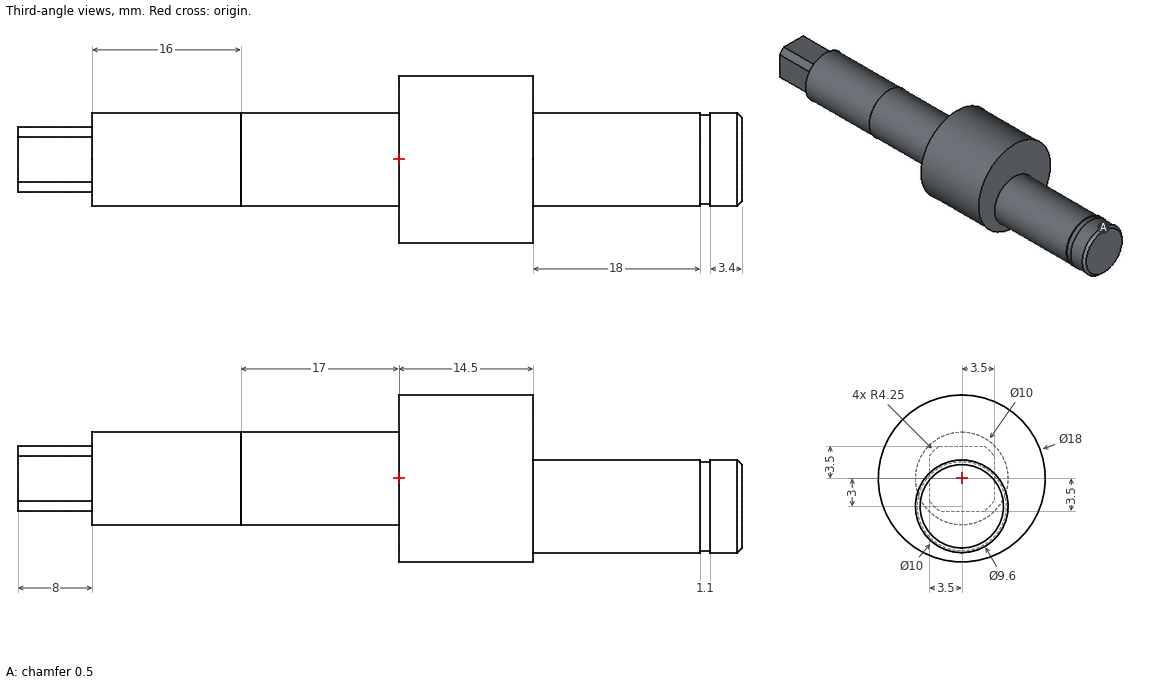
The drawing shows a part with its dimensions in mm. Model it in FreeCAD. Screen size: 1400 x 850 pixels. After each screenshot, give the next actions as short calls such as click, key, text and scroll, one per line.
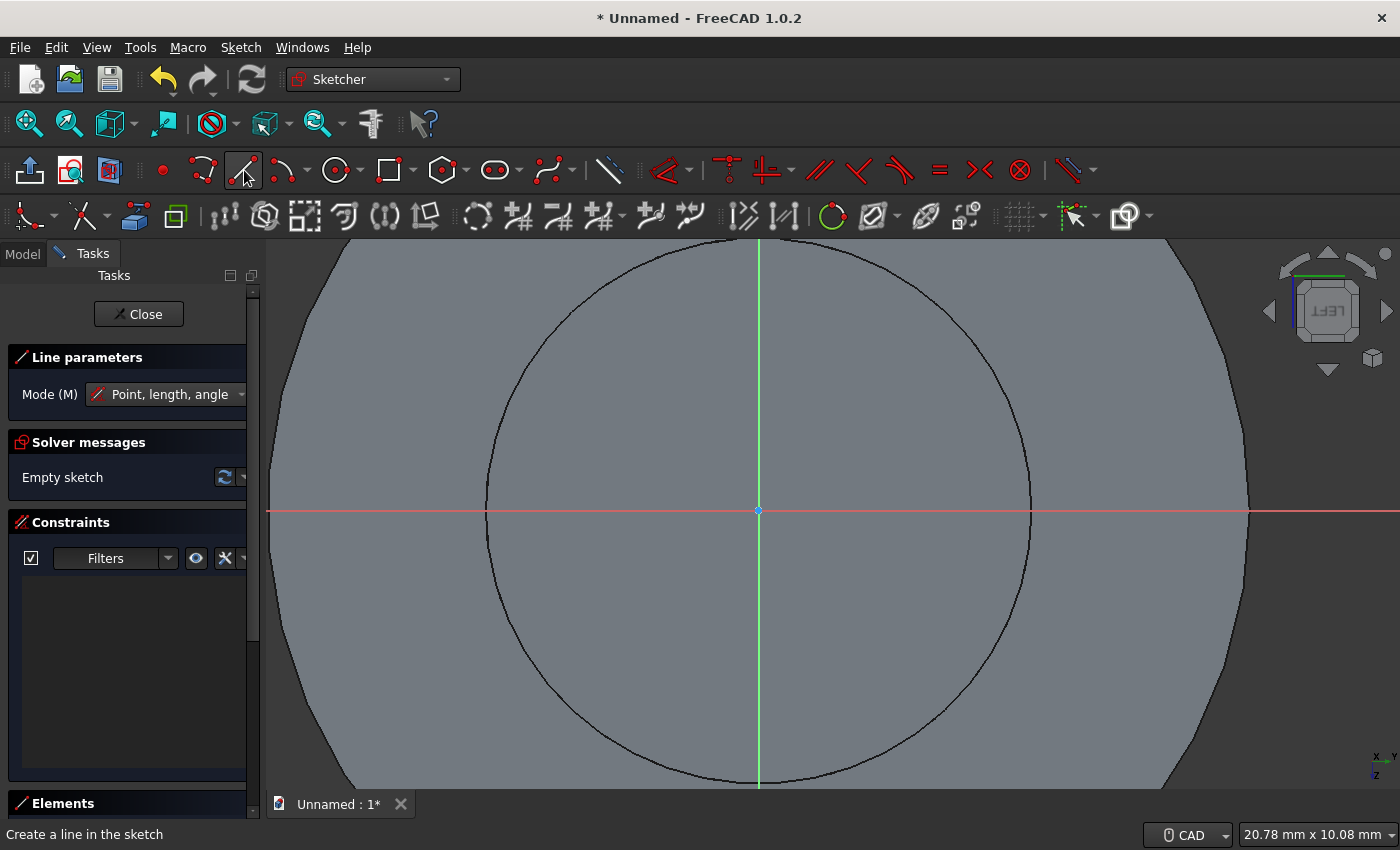
click(568, 379)
click(568, 642)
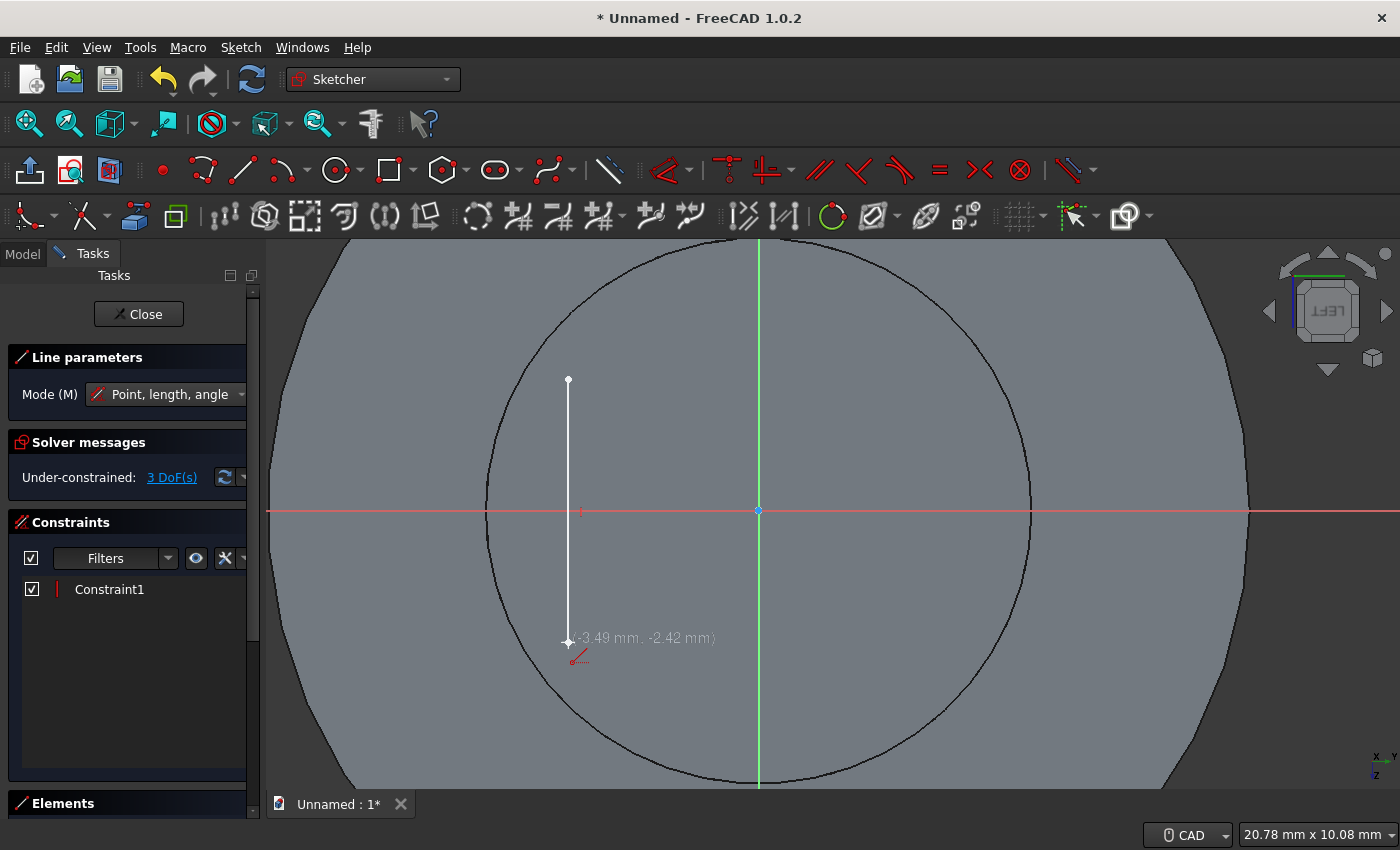
click(627, 702)
click(890, 702)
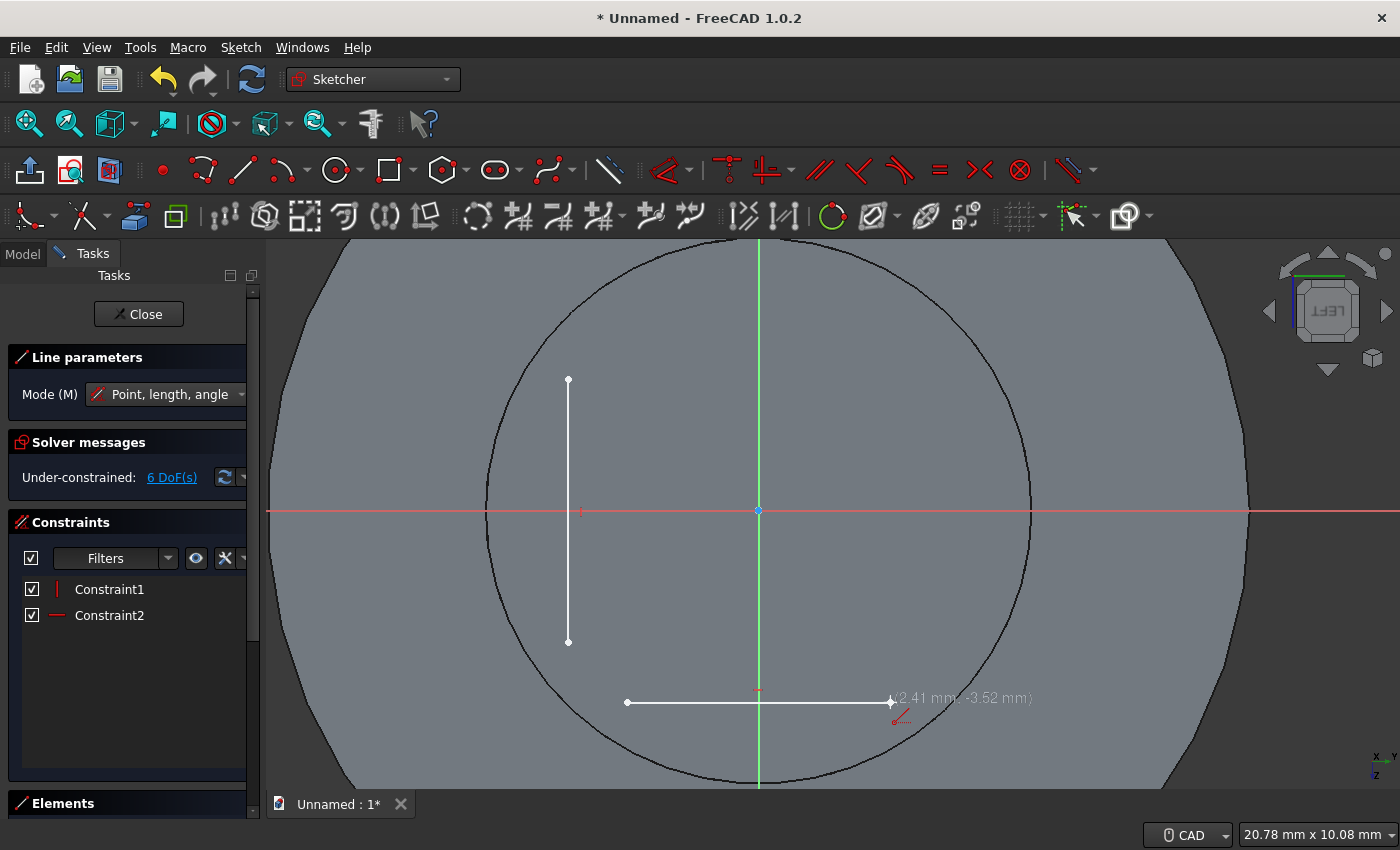
click(950, 642)
click(950, 379)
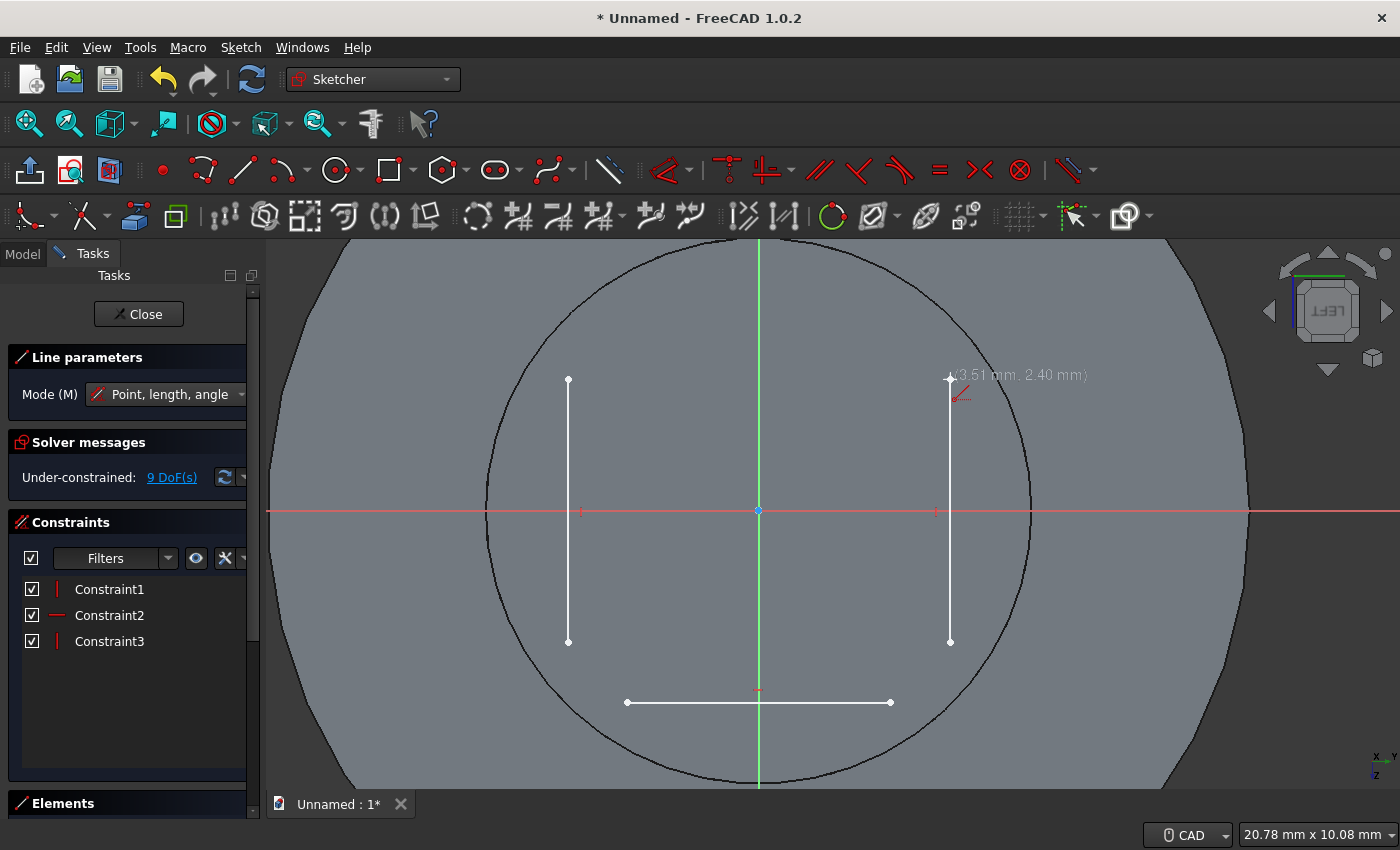
click(890, 320)
click(627, 320)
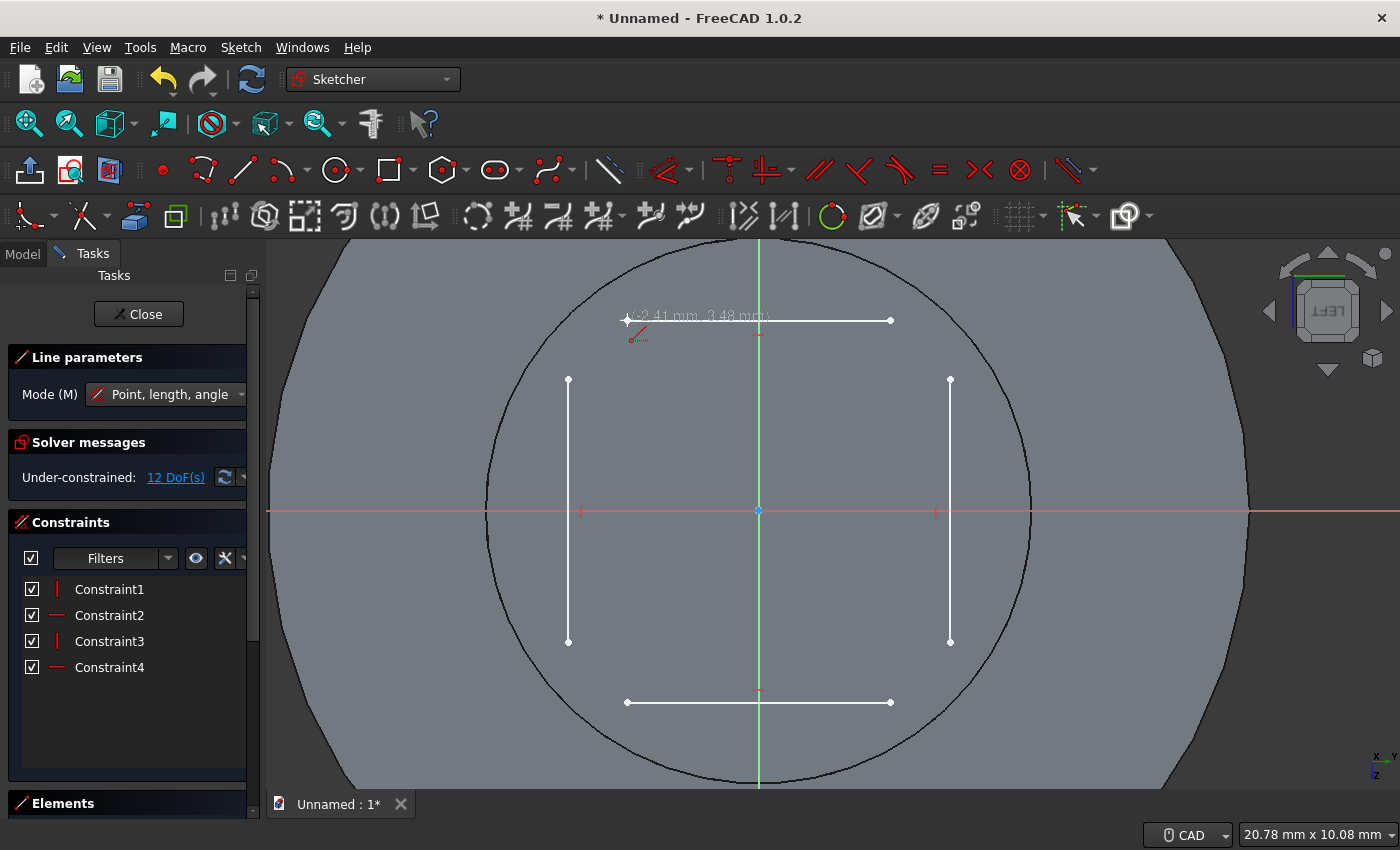
click(310, 170)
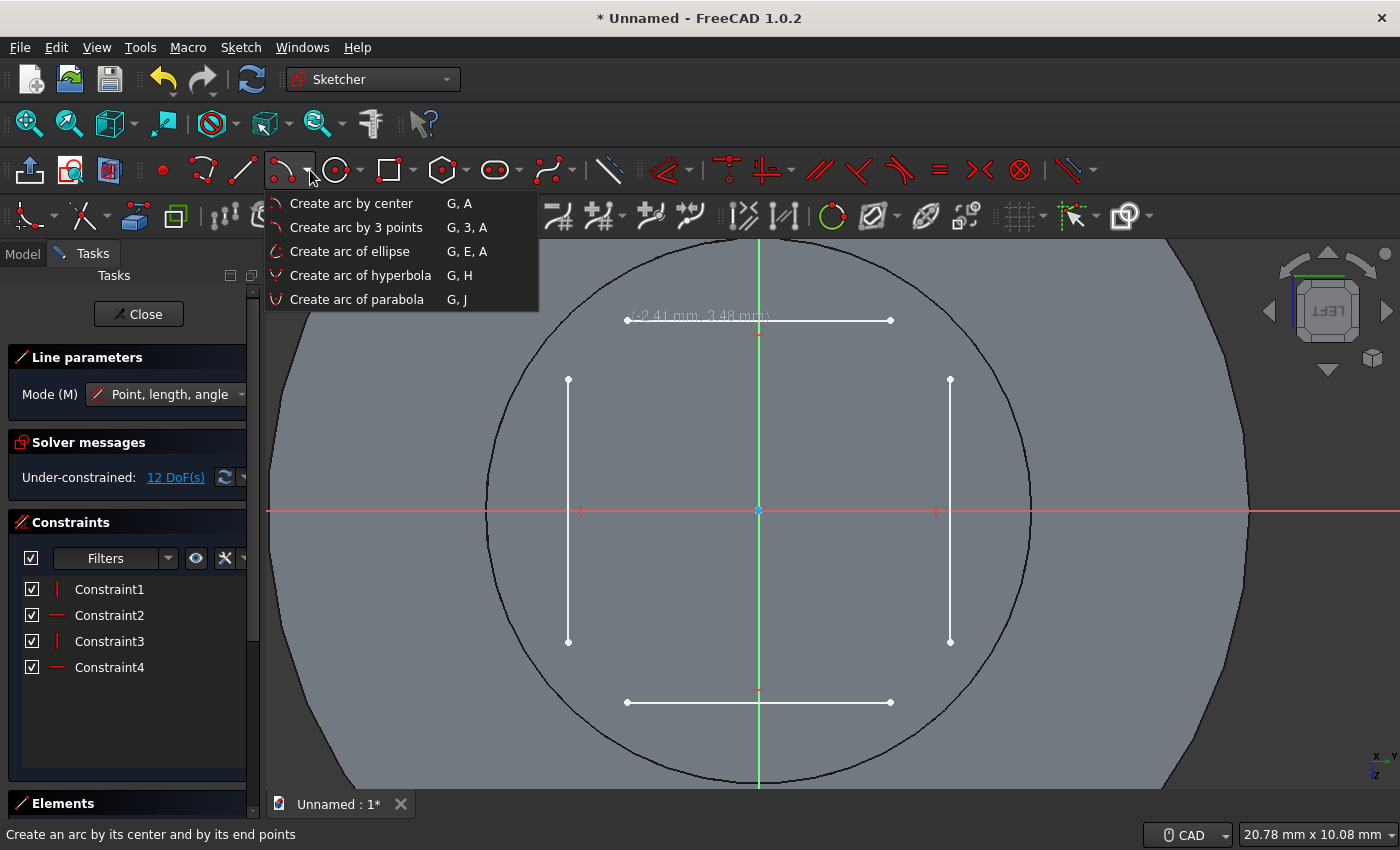
click(402, 227)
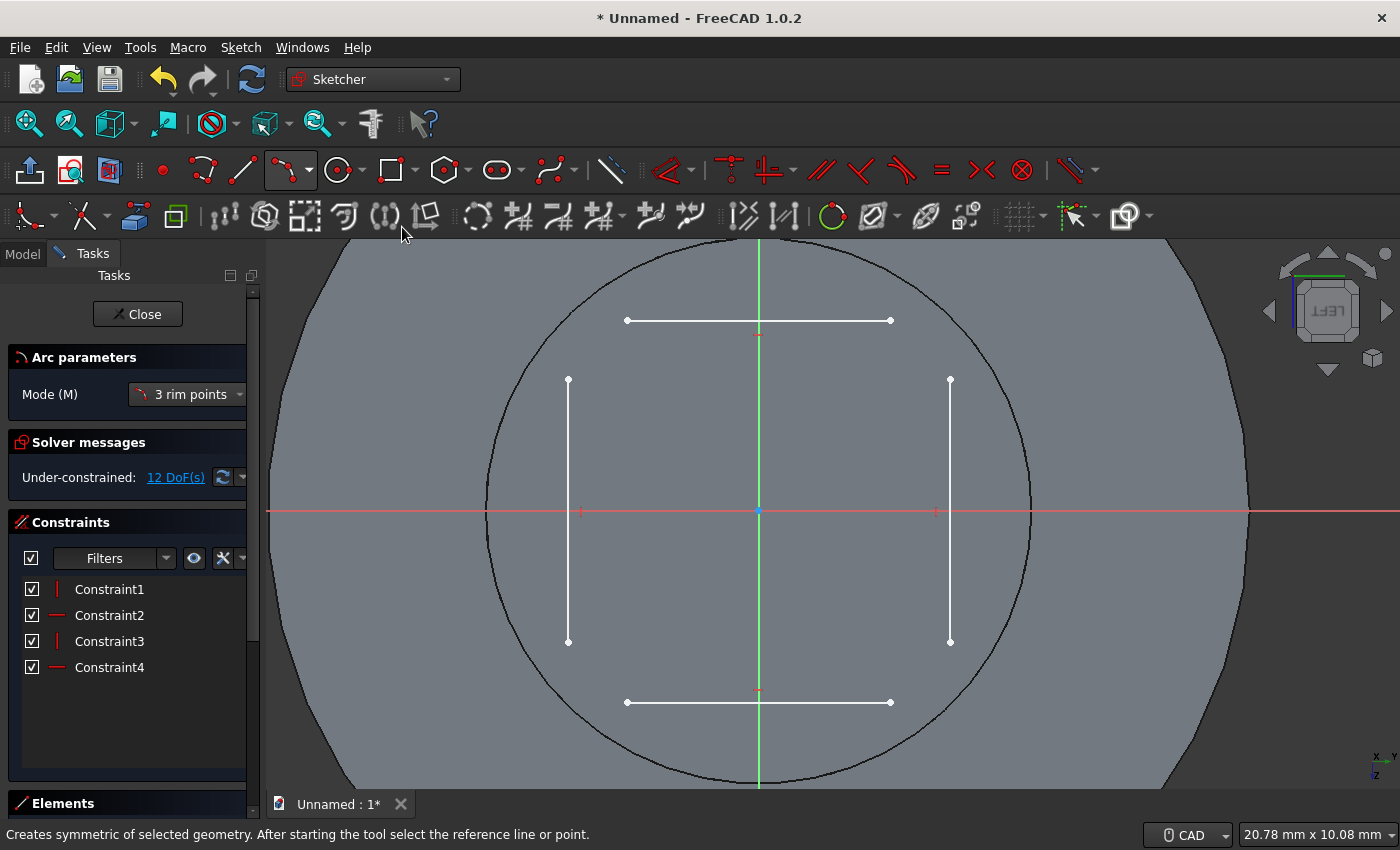
click(568, 643)
click(627, 703)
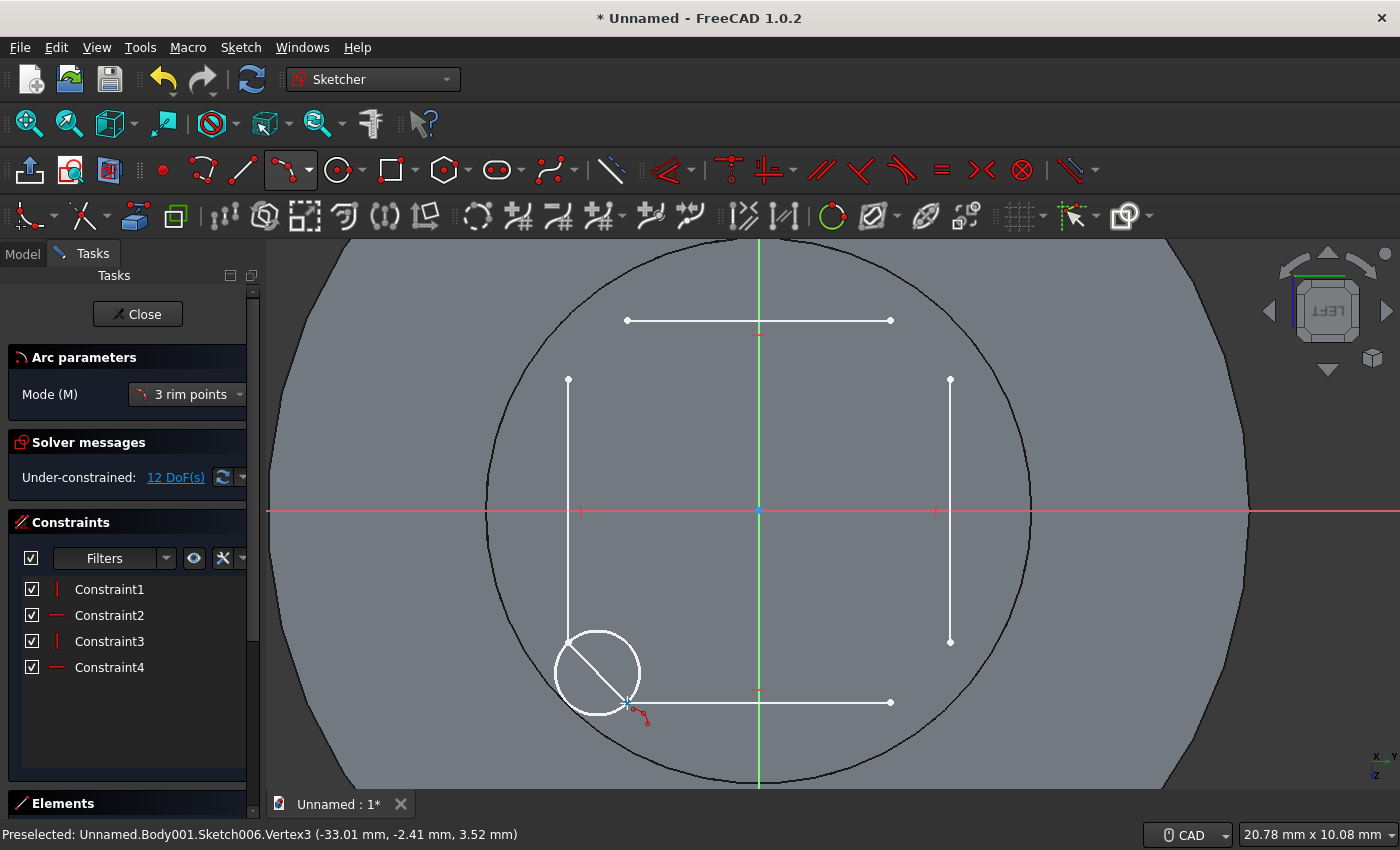
scroll(595, 675, up, 8)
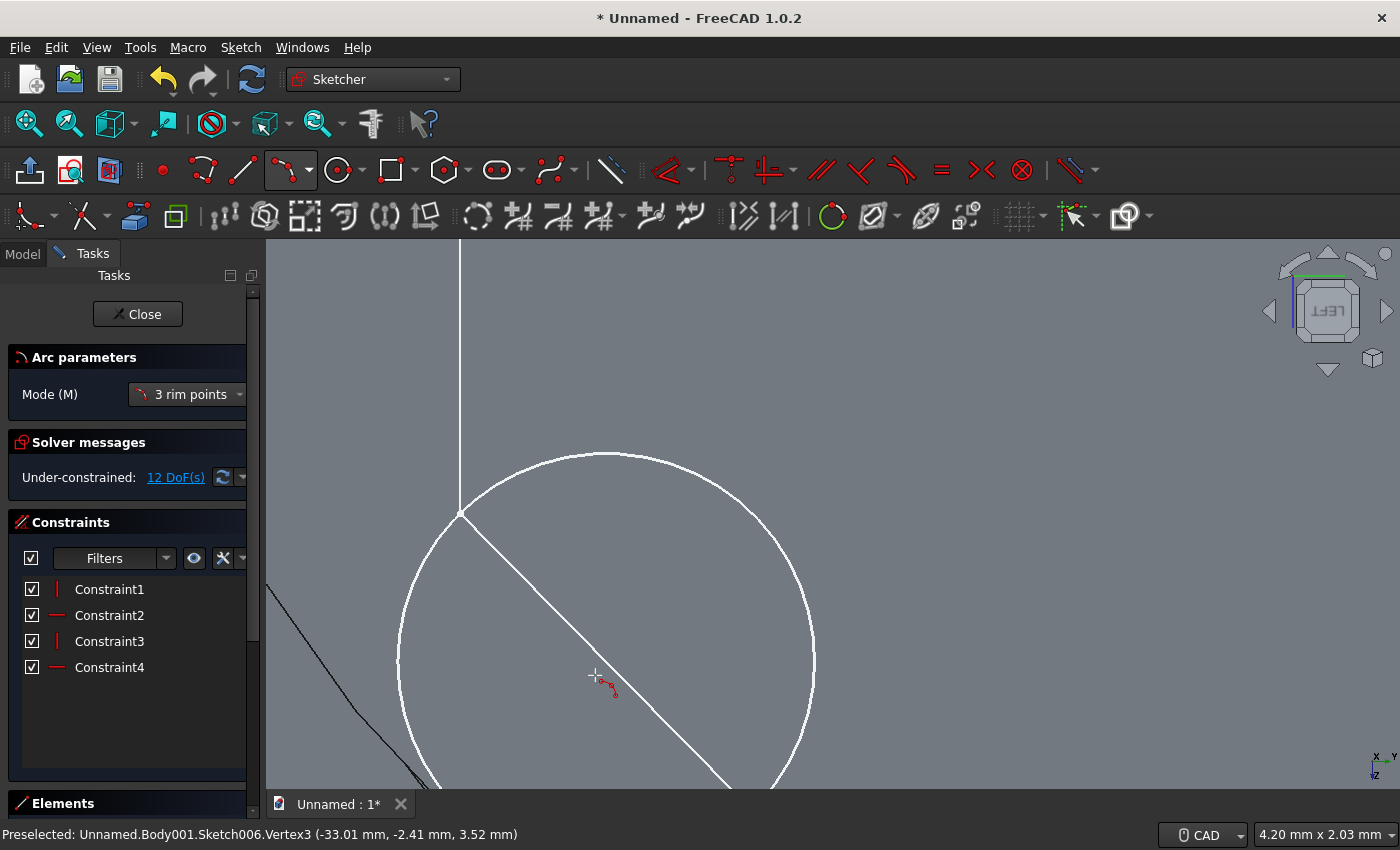
click(592, 671)